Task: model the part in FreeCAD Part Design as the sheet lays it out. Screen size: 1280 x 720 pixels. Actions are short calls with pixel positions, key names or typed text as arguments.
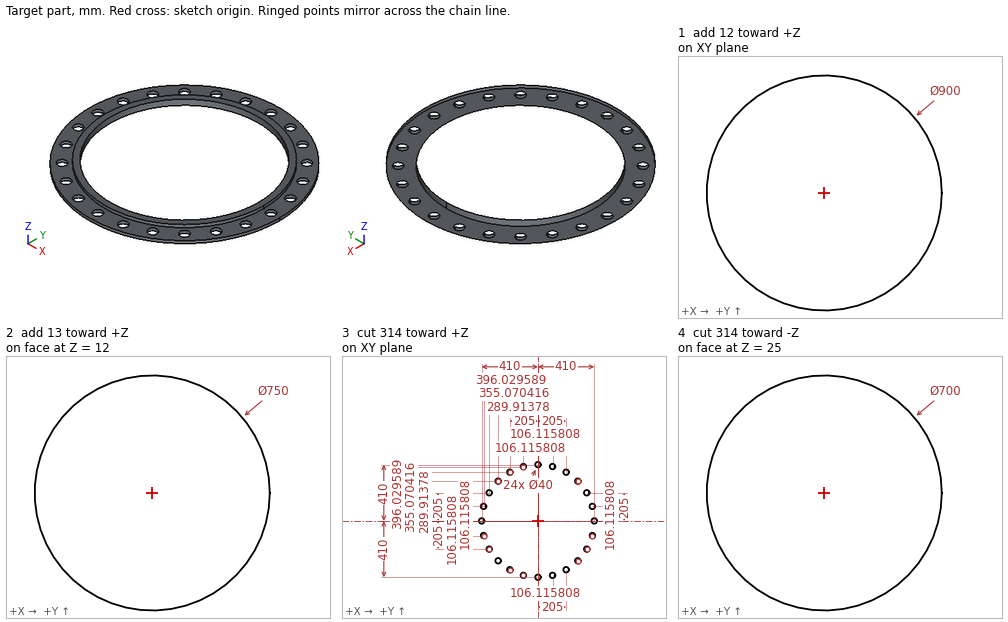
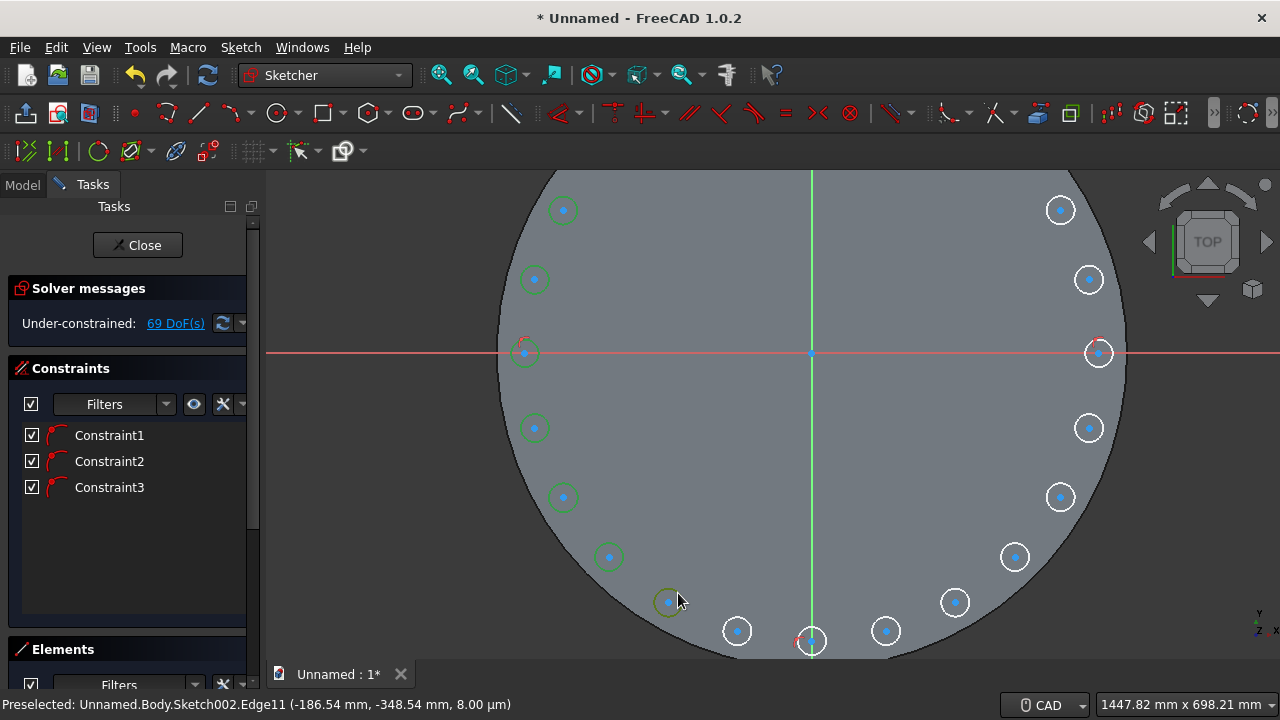
click(747, 621)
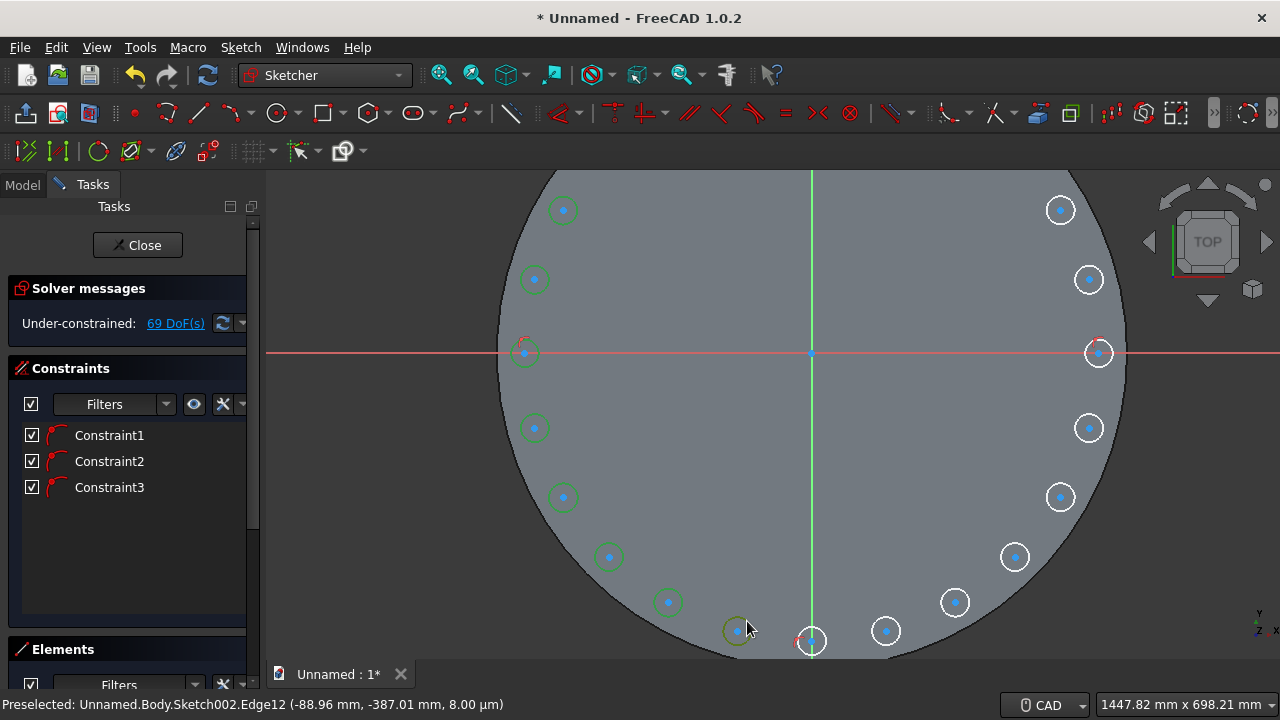
click(812, 627)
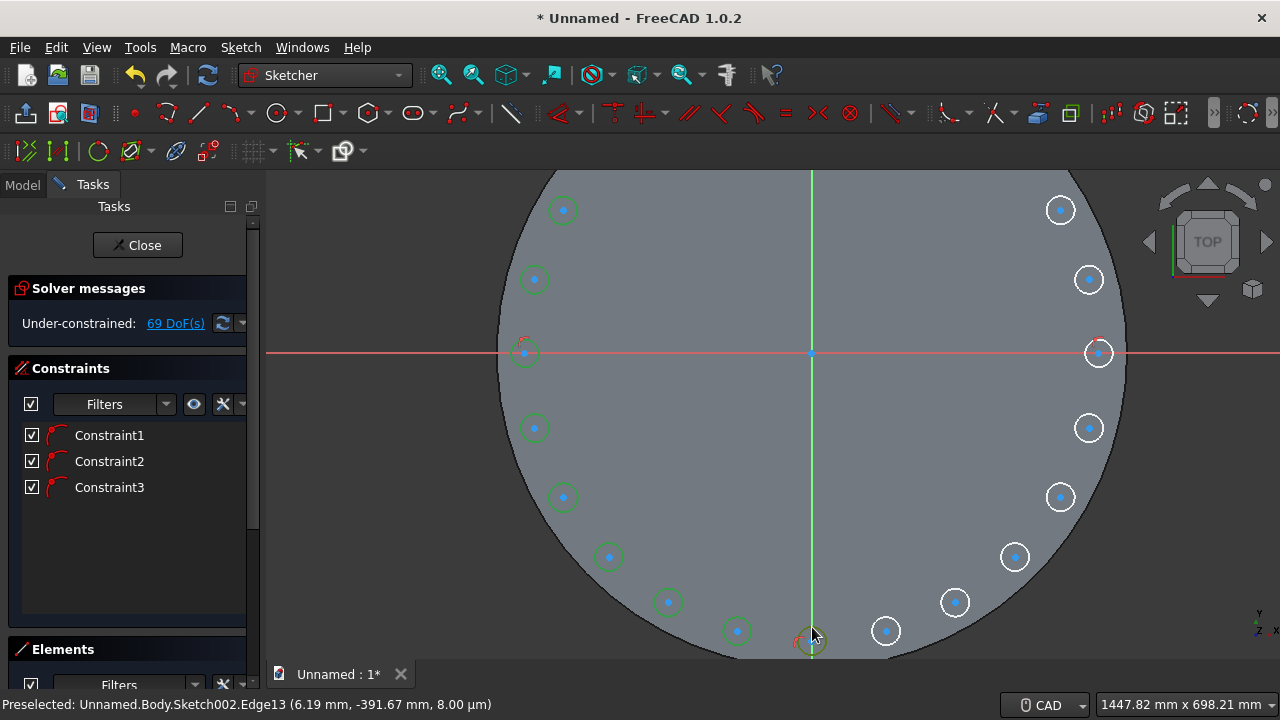
click(896, 621)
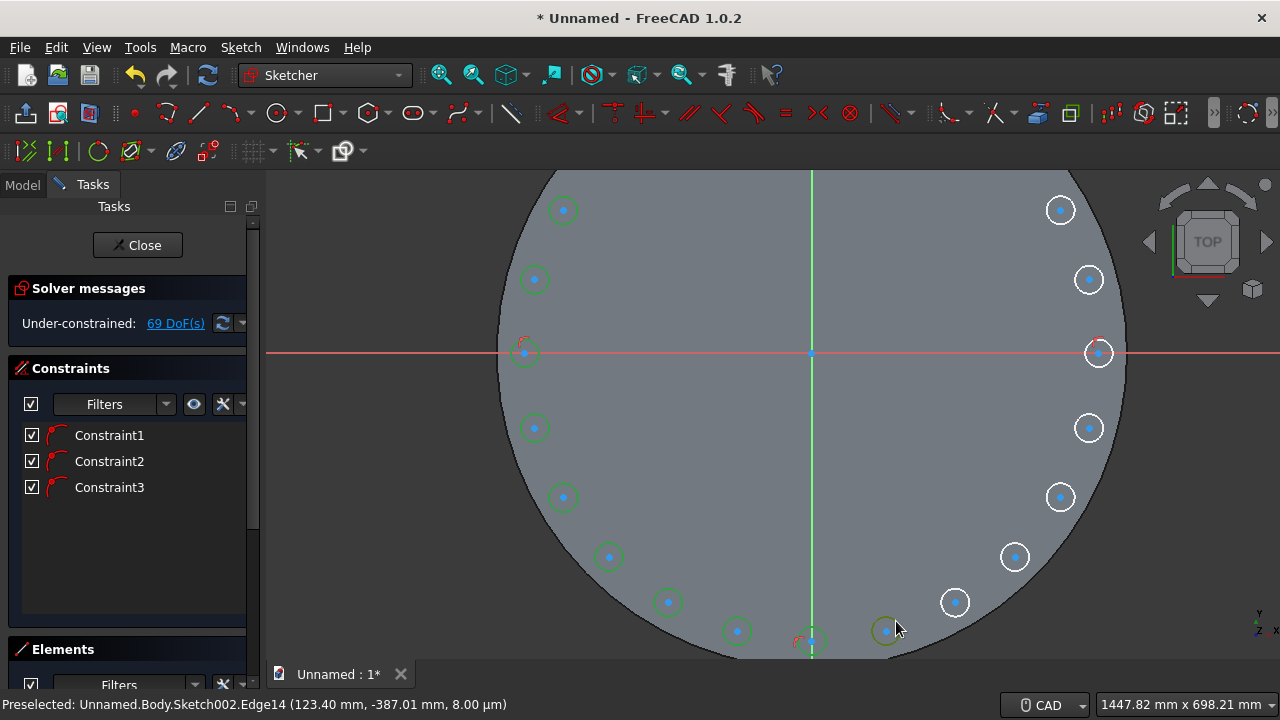
click(965, 593)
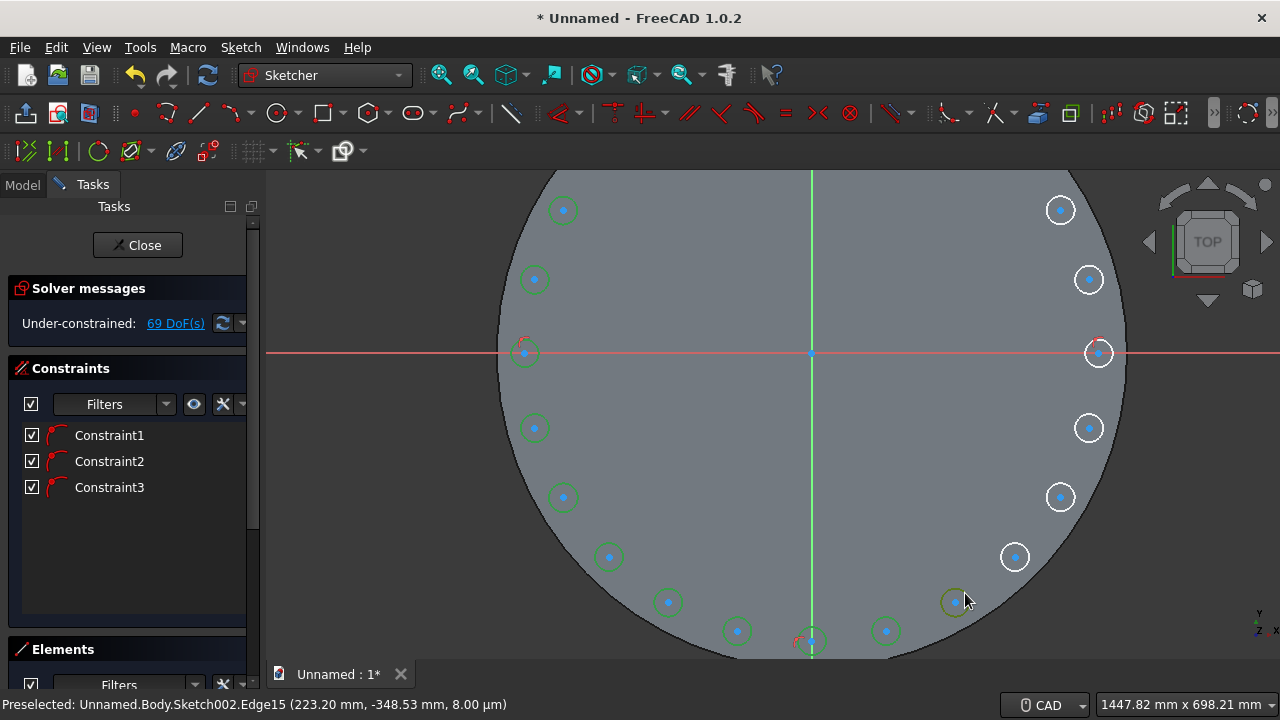
click(1025, 547)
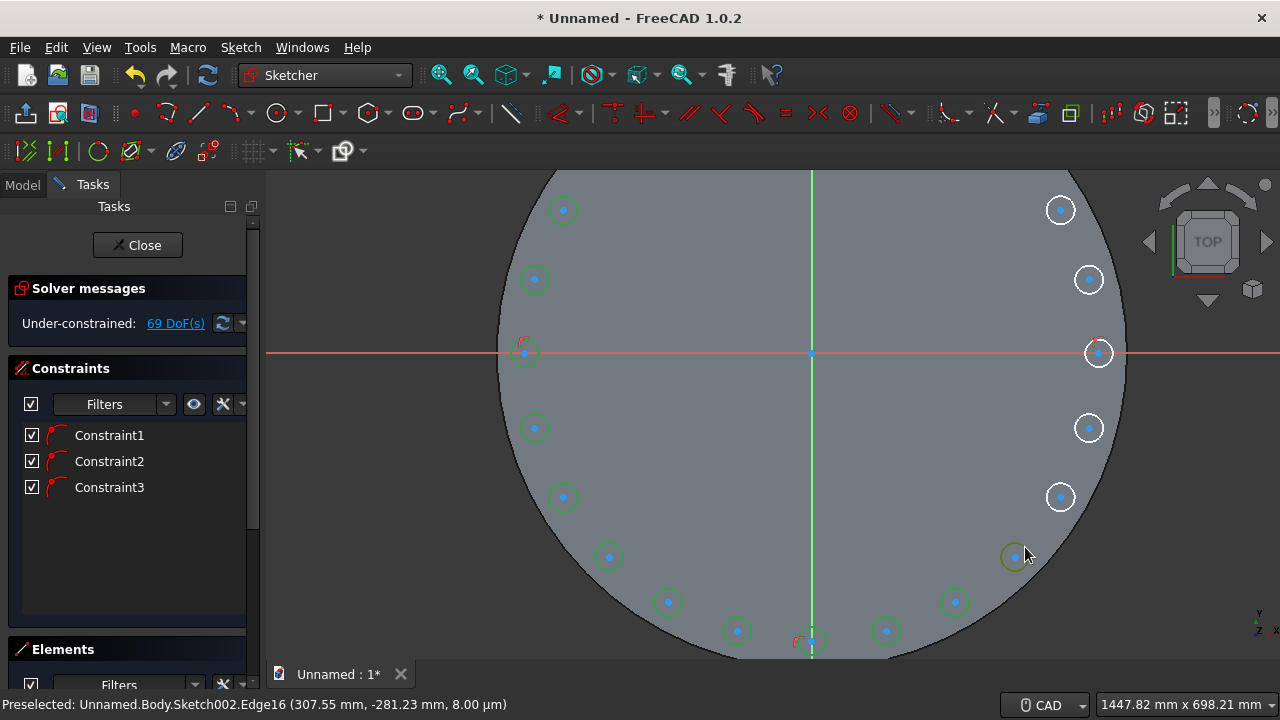
click(1070, 487)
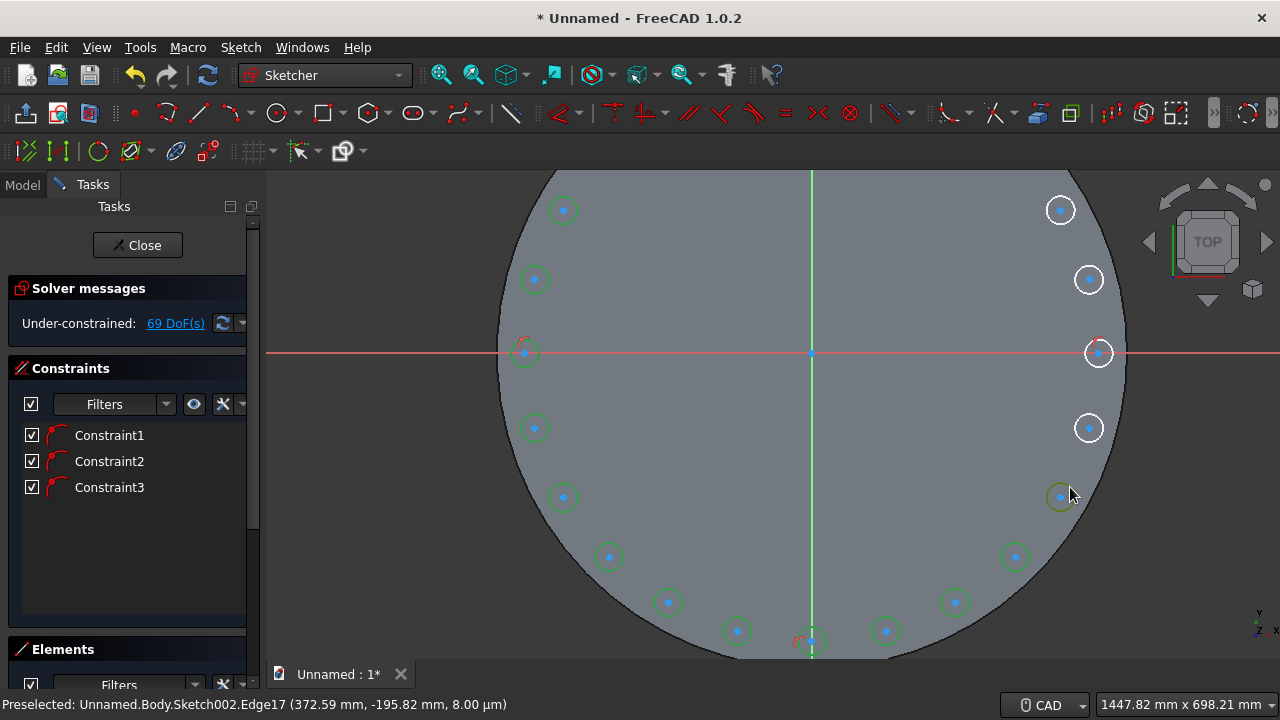
click(1099, 418)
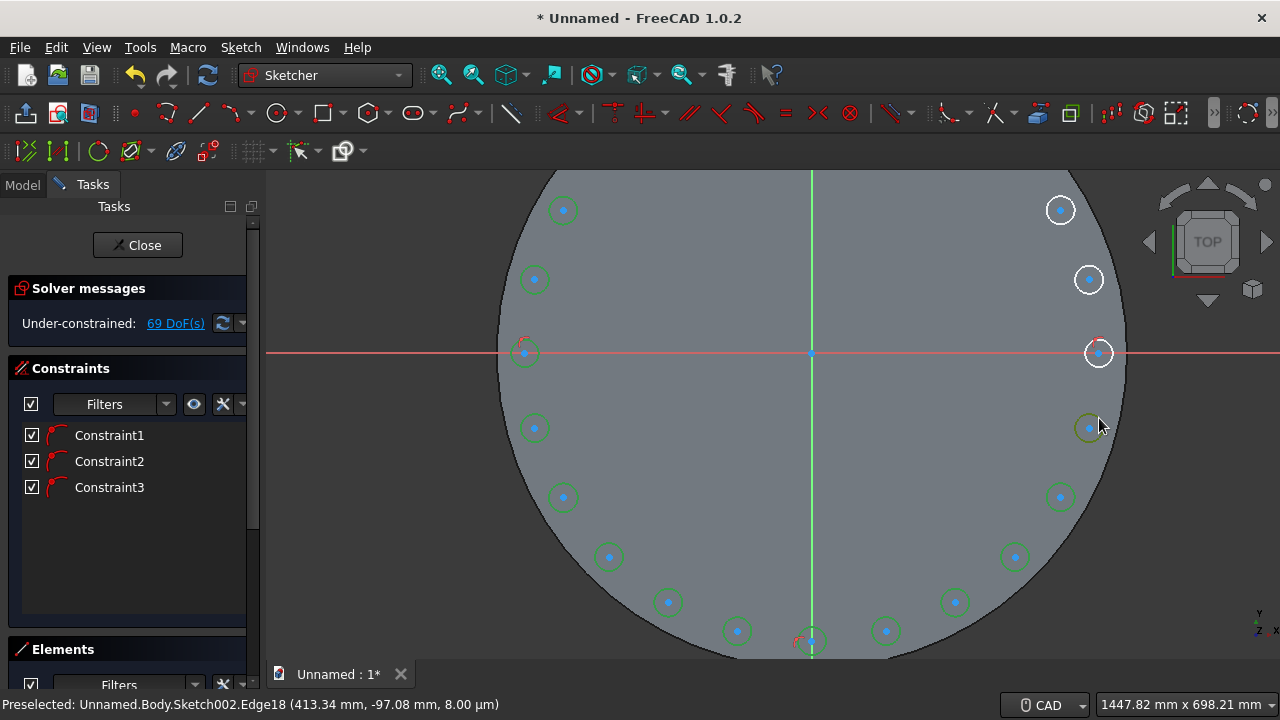
scroll(1109, 344, up, 2)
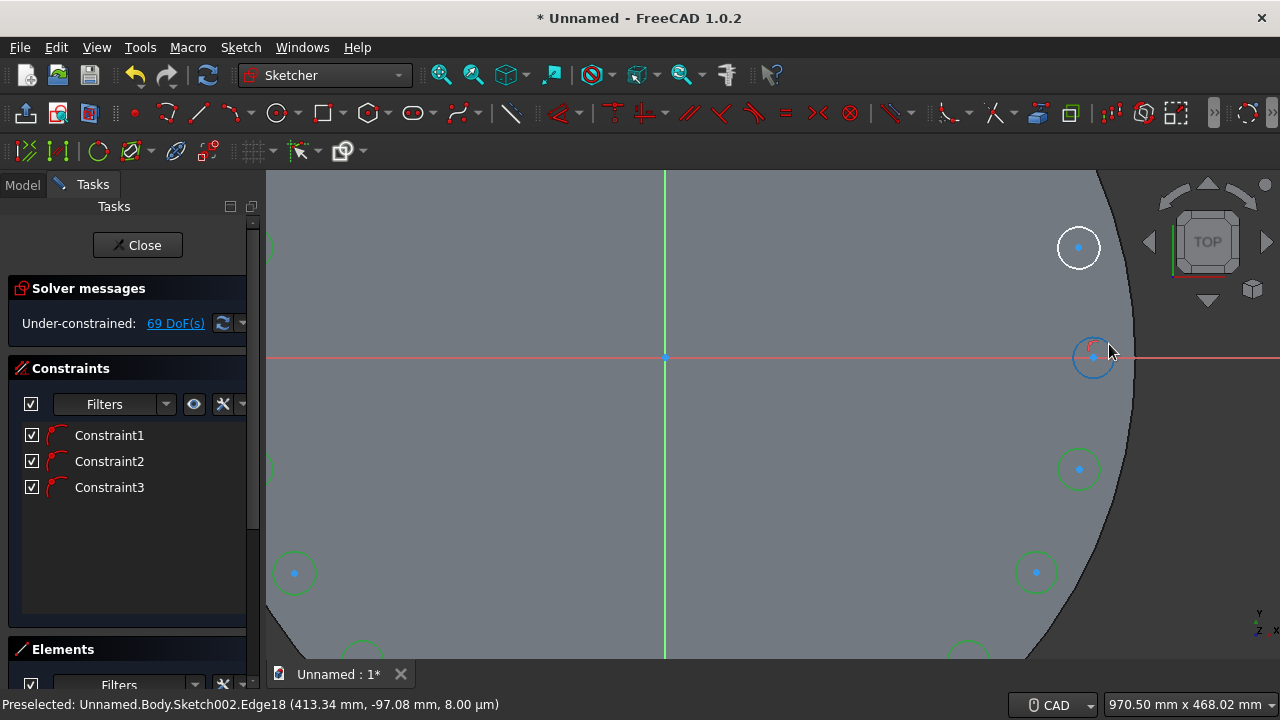
click(1108, 343)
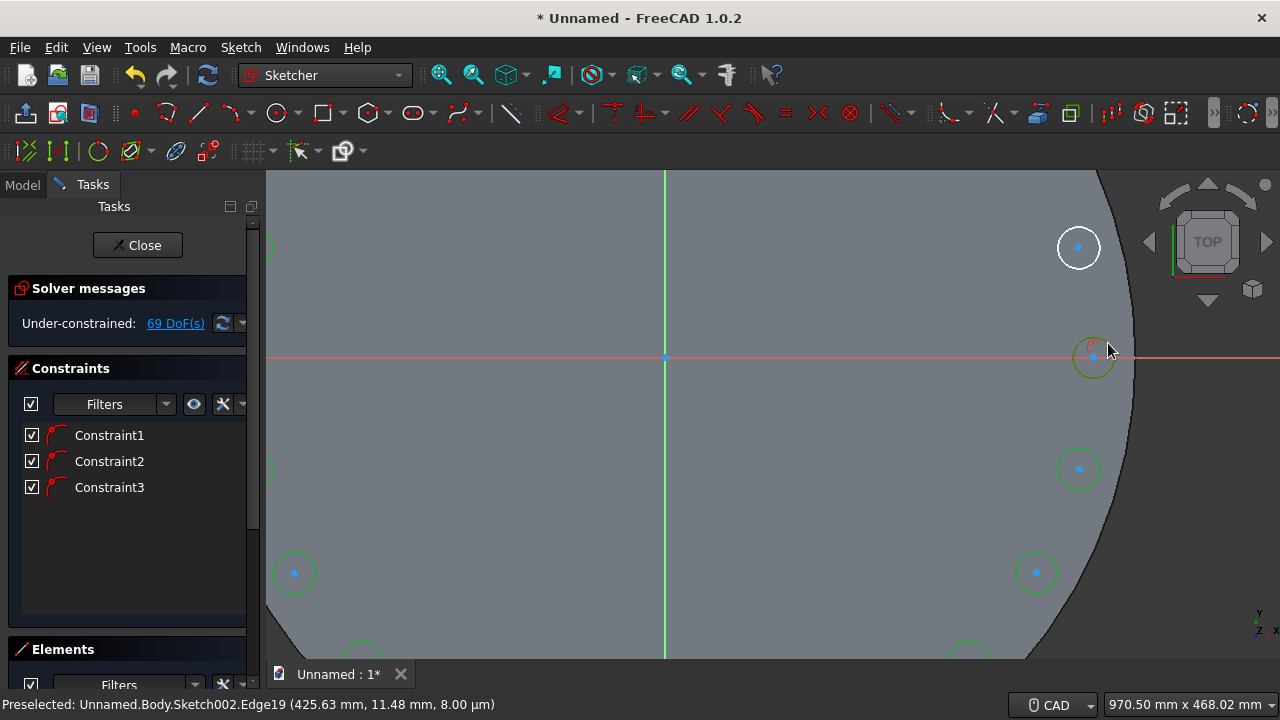
click(1094, 233)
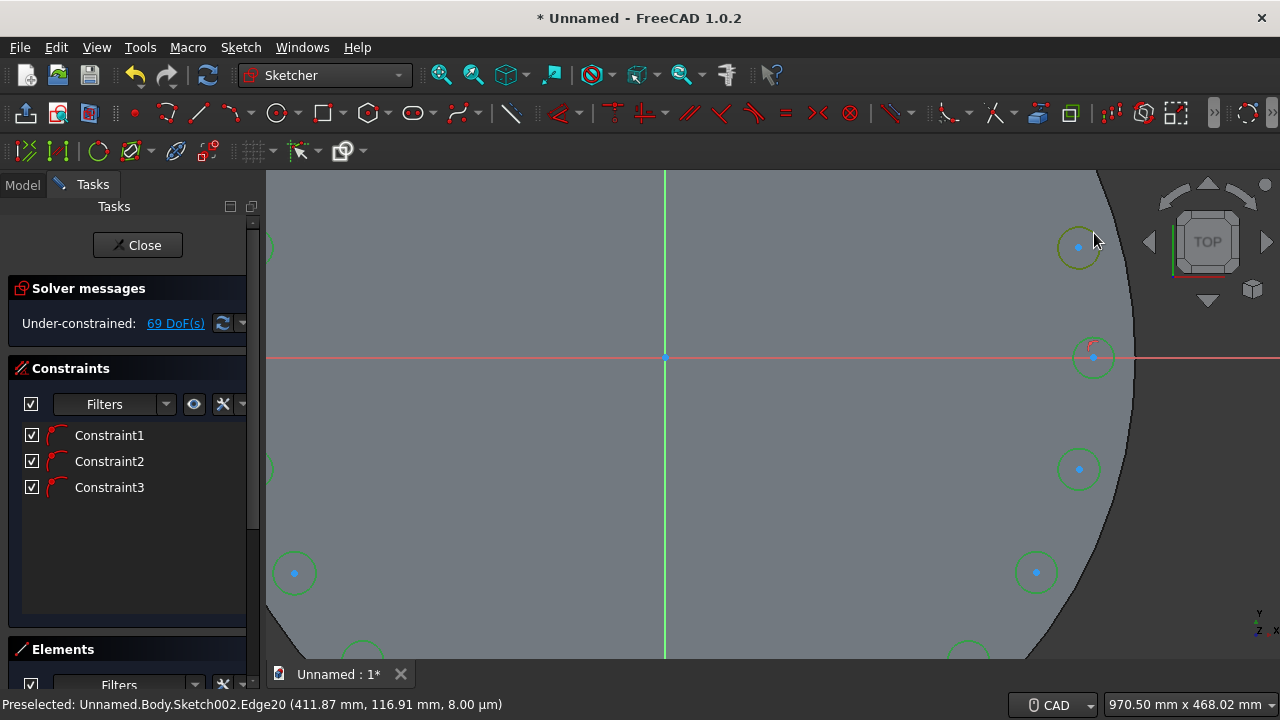
scroll(727, 447, down, 5)